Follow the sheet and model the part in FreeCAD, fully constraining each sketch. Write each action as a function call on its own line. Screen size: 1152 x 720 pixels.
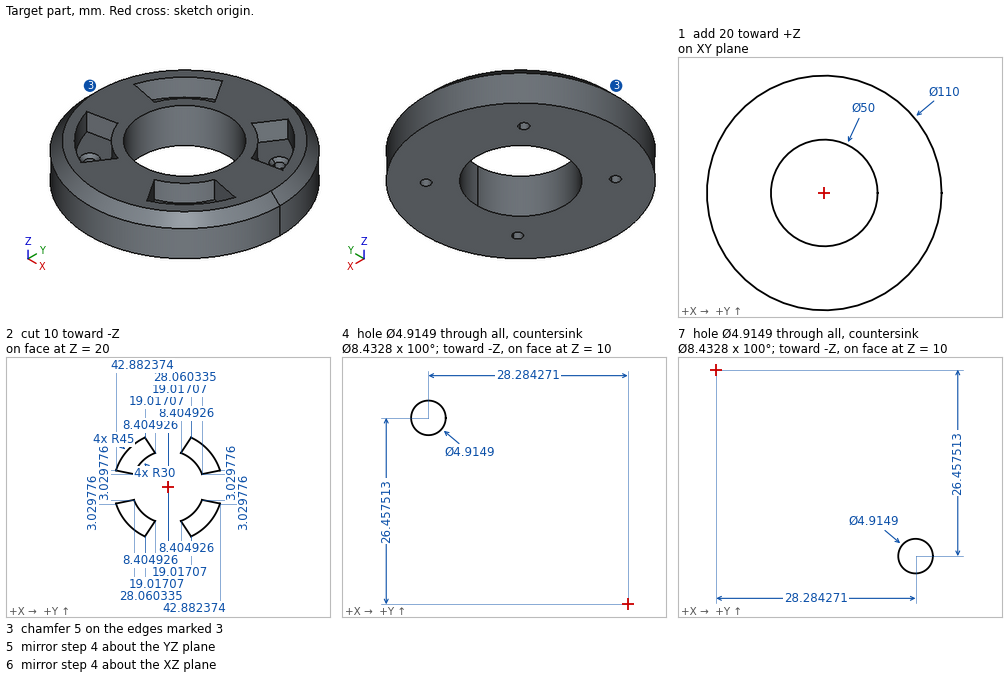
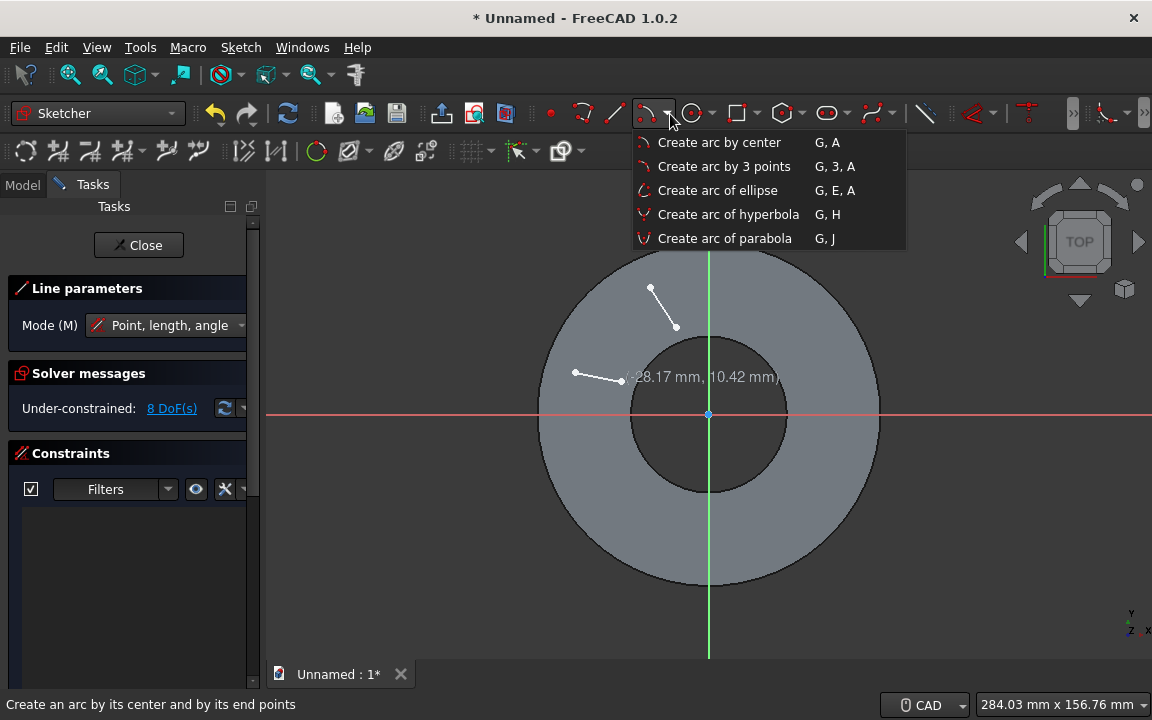
click(770, 166)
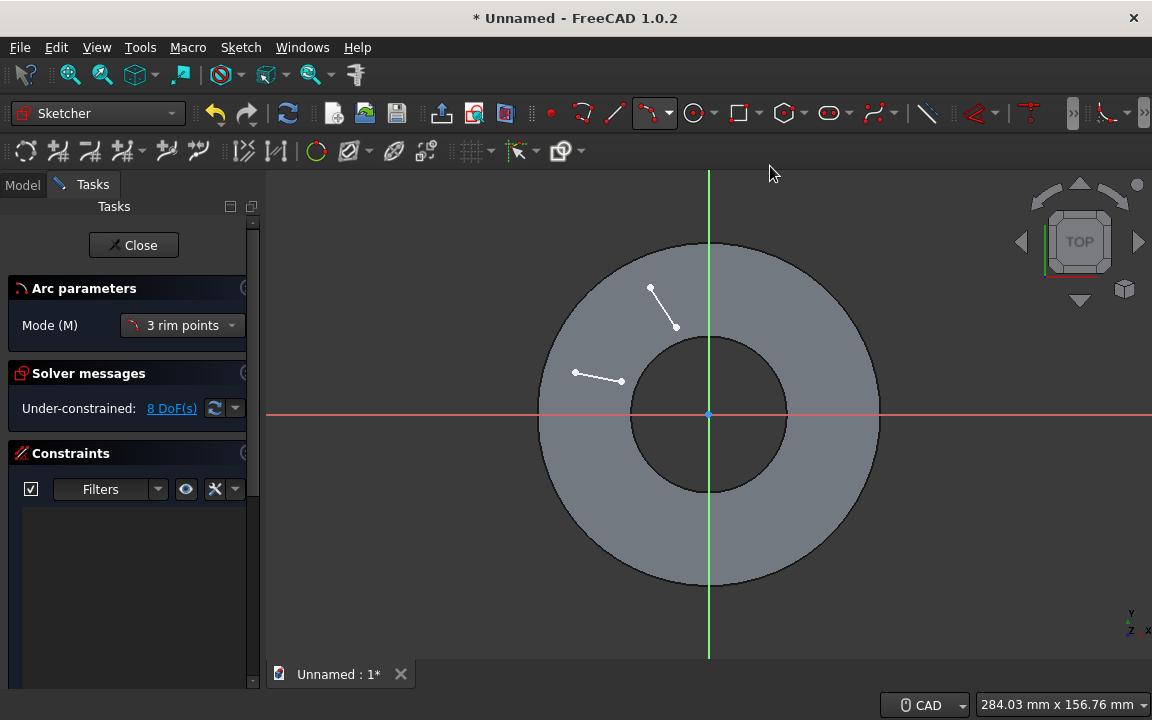
click(650, 288)
click(575, 373)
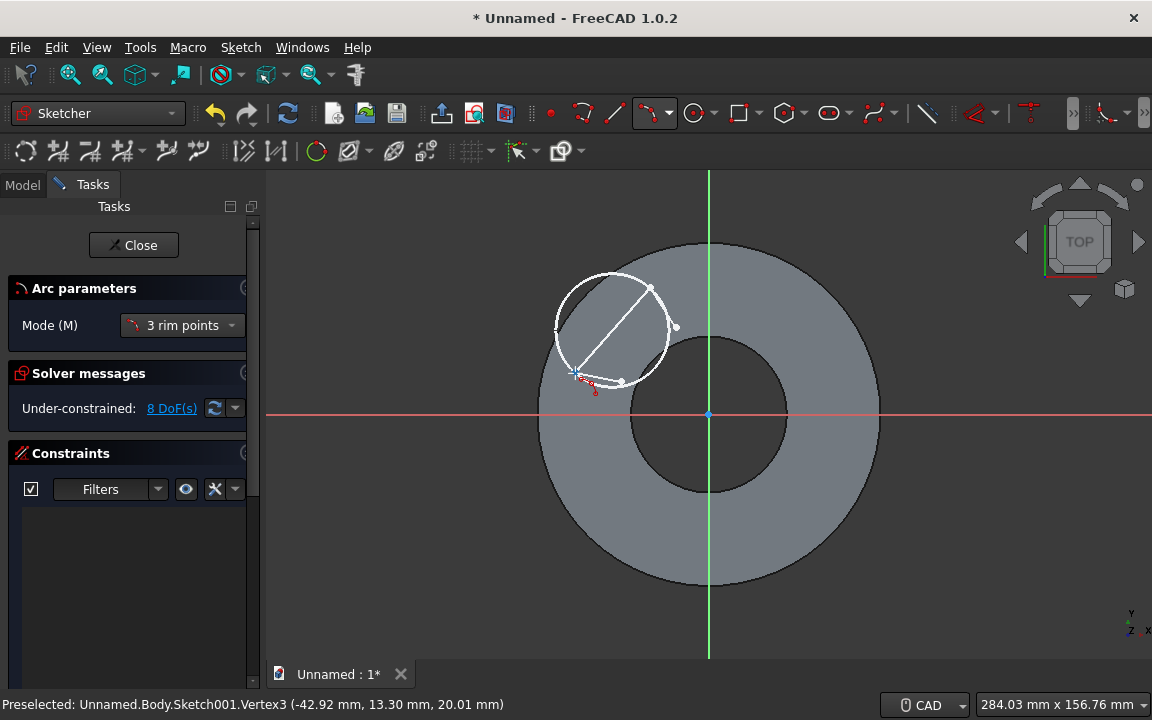
scroll(603, 322, up, 2)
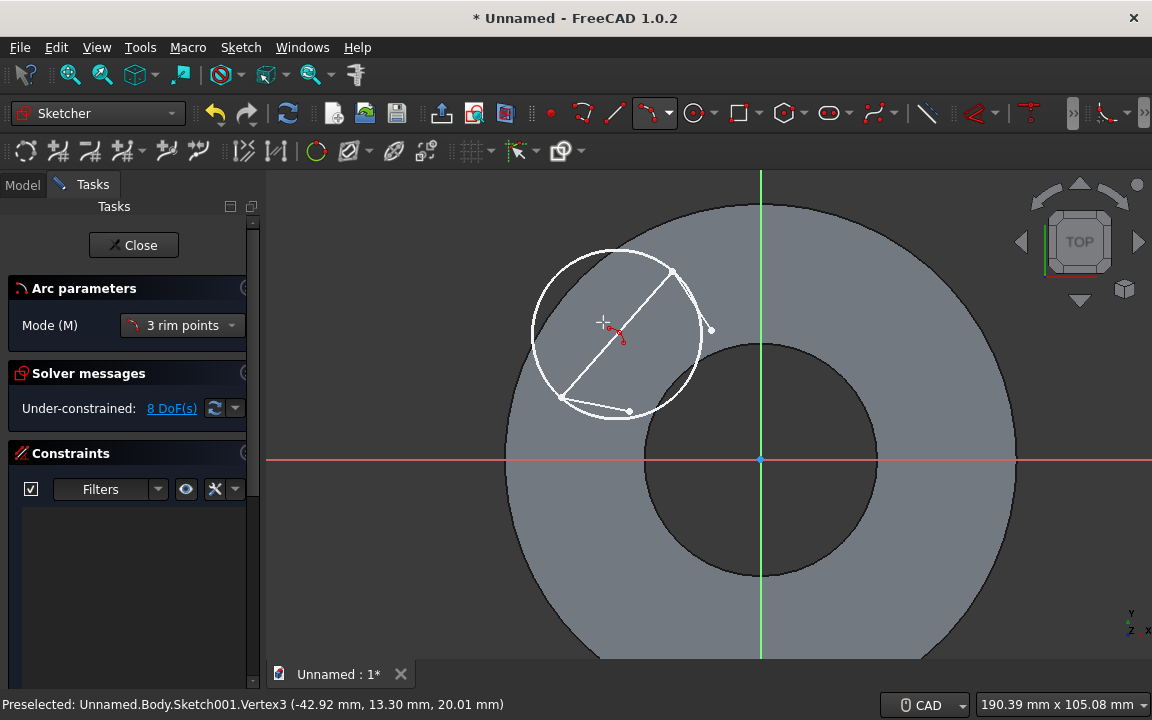
click(604, 322)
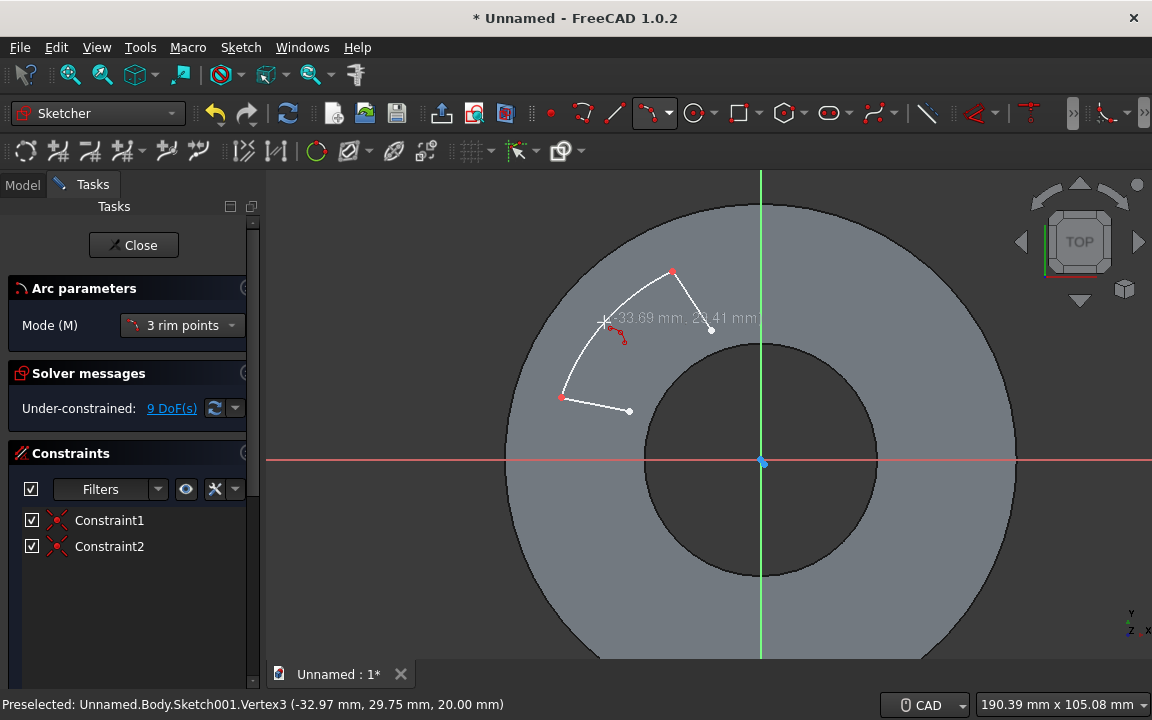
click(630, 411)
click(712, 331)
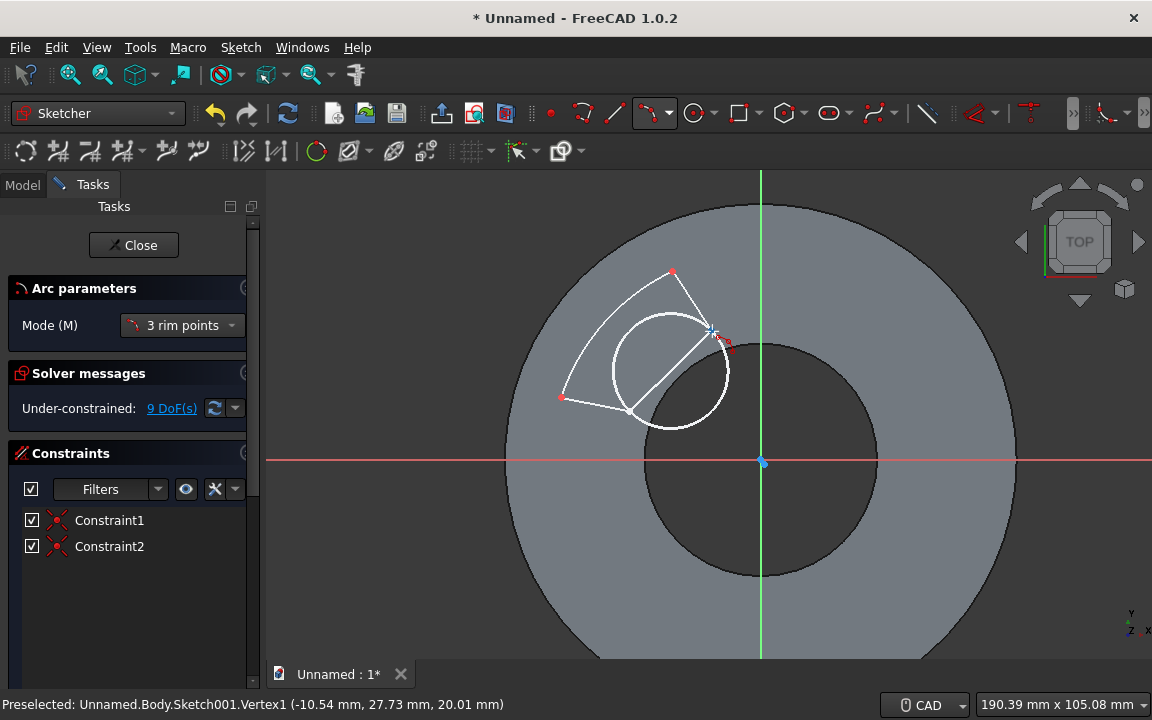
scroll(662, 361, up, 2)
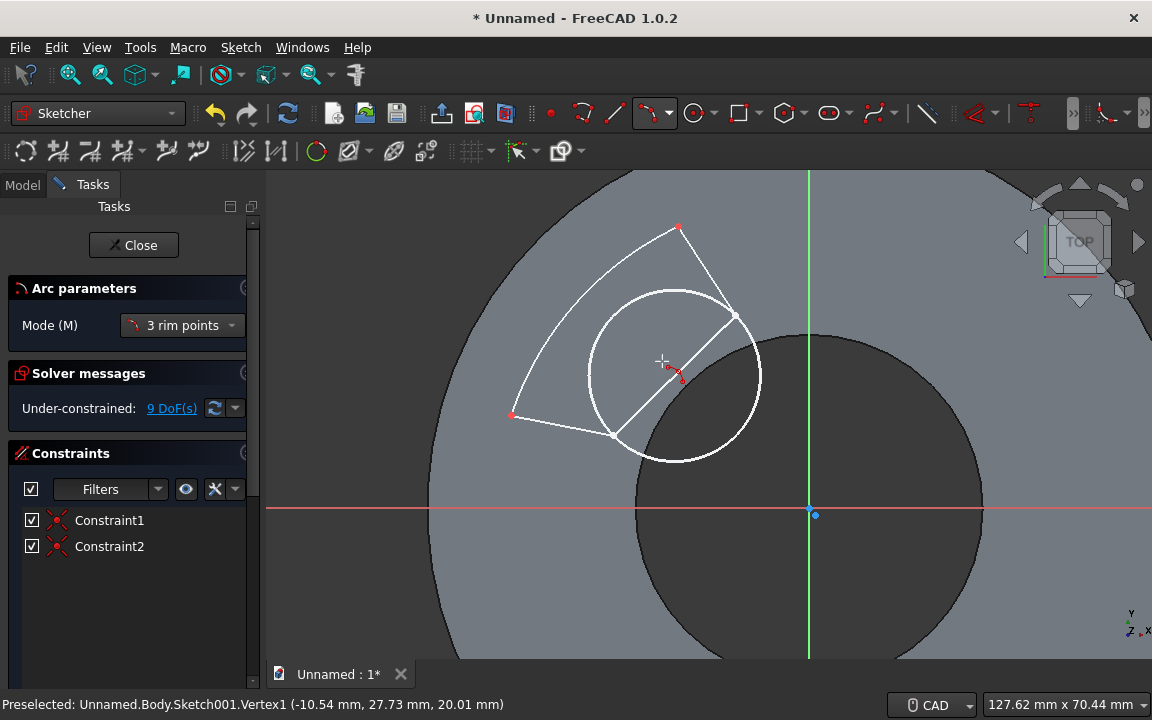
click(662, 361)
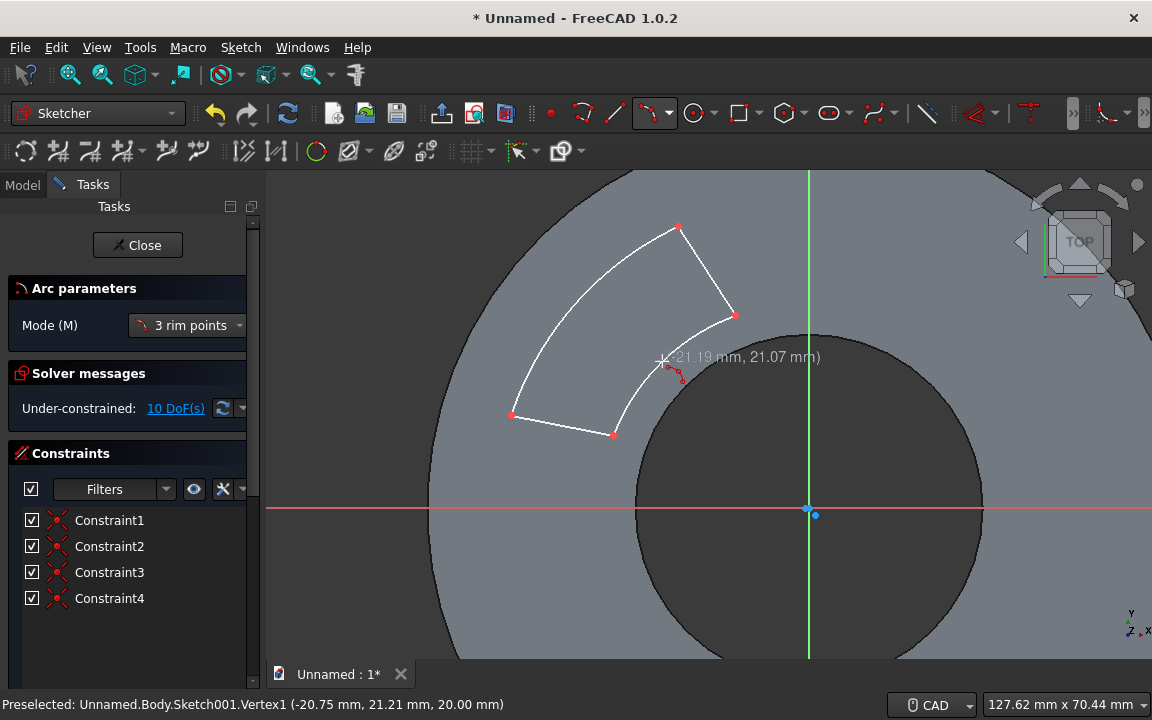
click(616, 114)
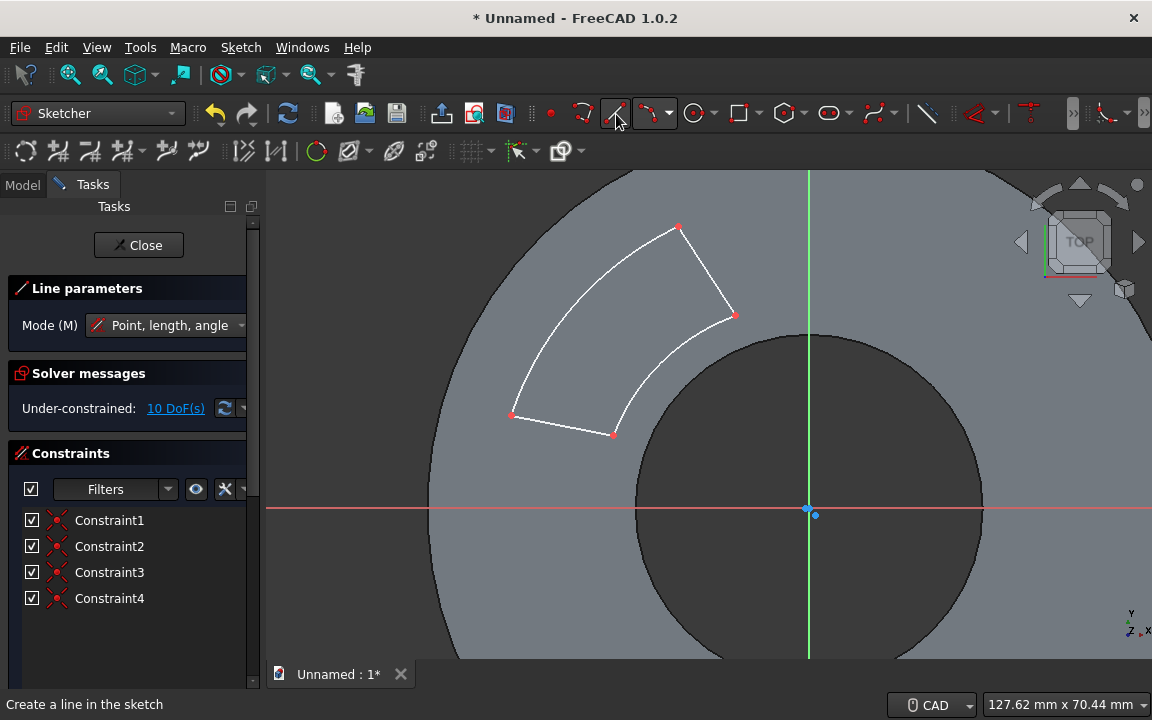
scroll(435, 300, down, 3)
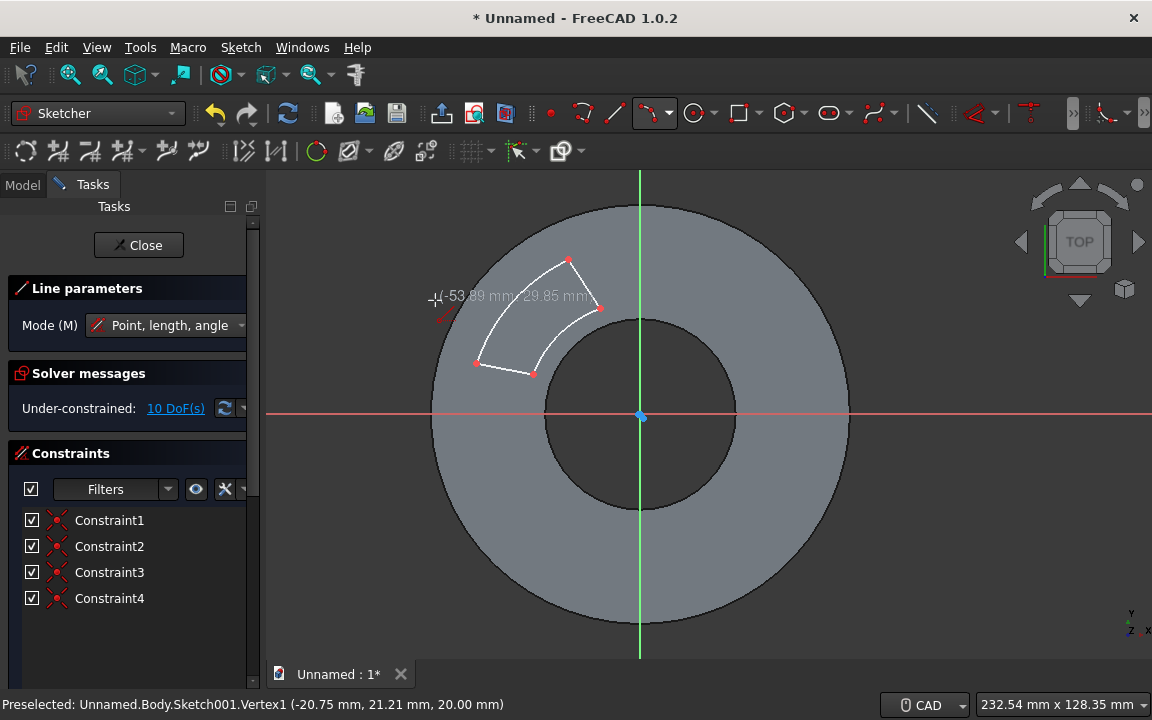
click(747, 374)
click(804, 362)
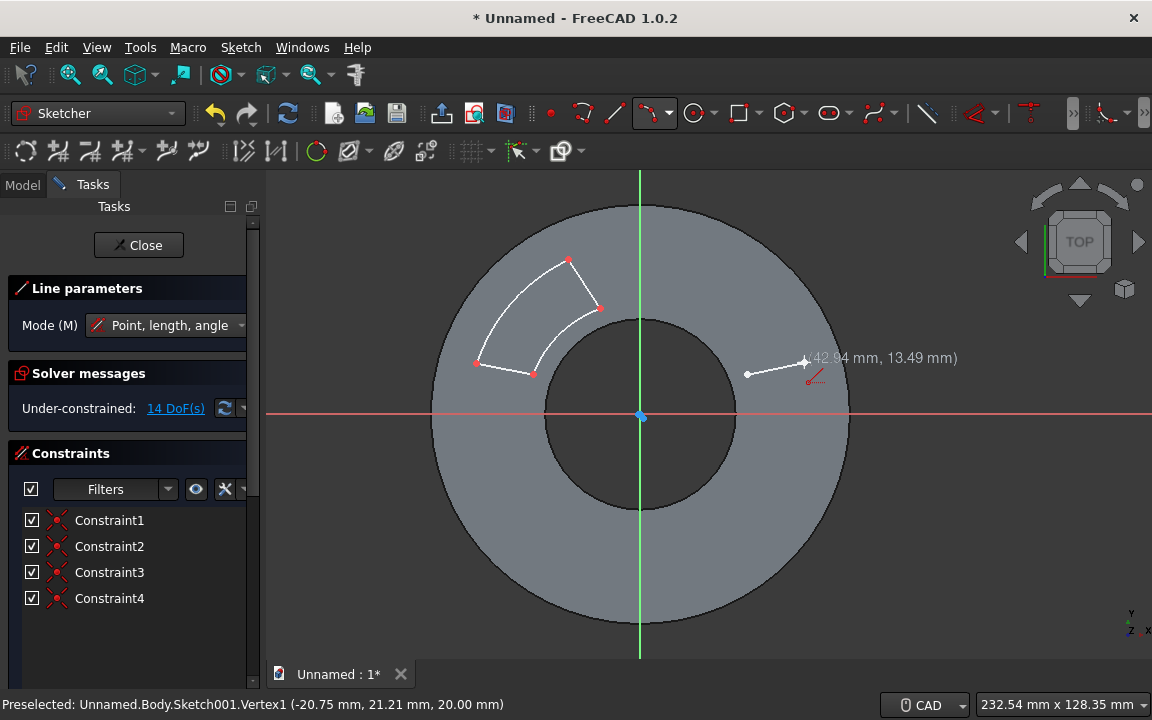
click(713, 259)
click(681, 308)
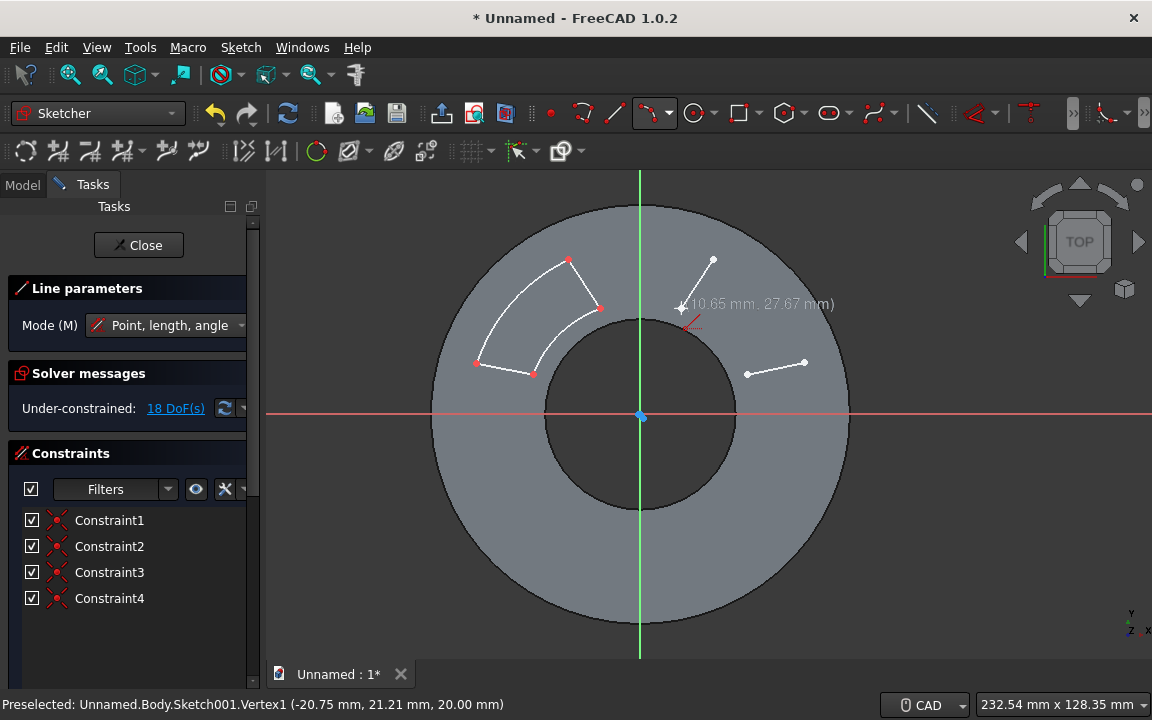
click(648, 114)